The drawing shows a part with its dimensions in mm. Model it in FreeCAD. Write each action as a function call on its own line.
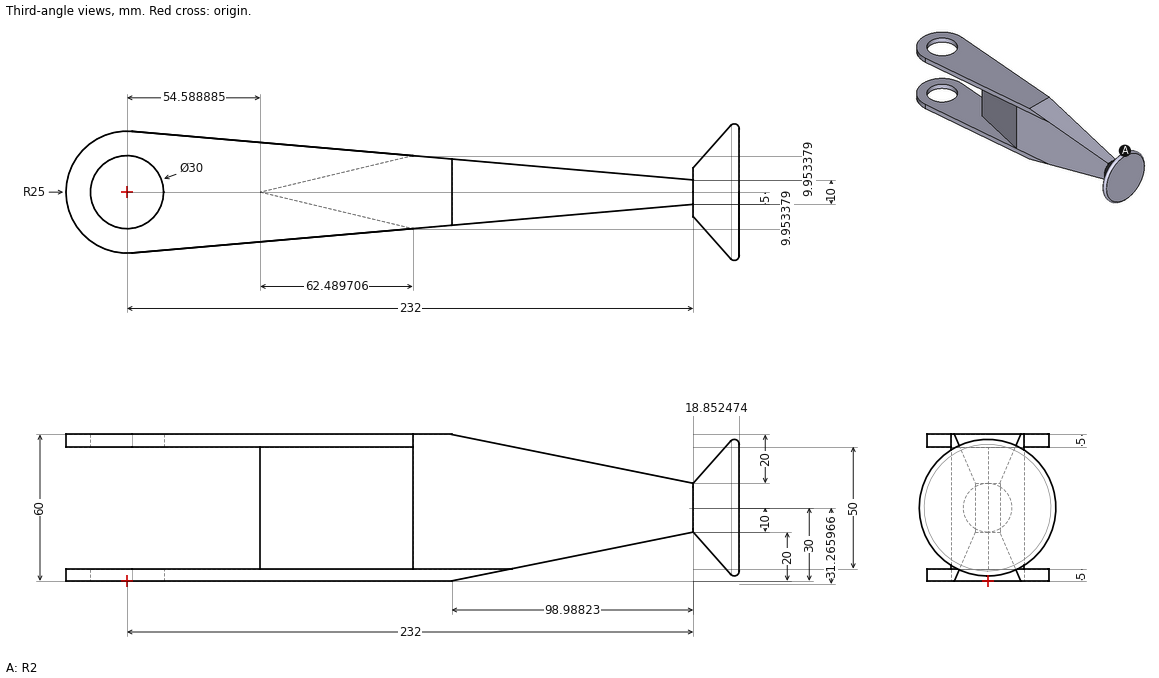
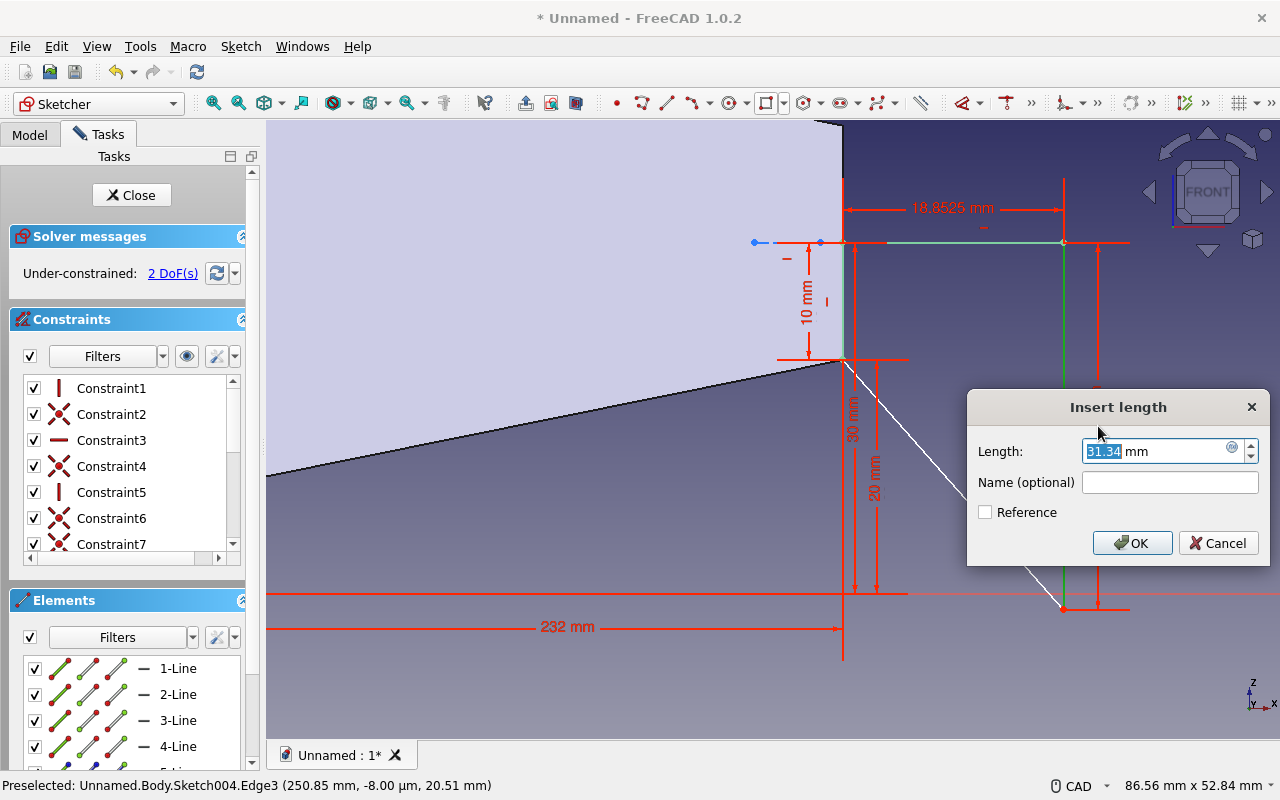
text(31.265966)
key(Return)
key(Escape)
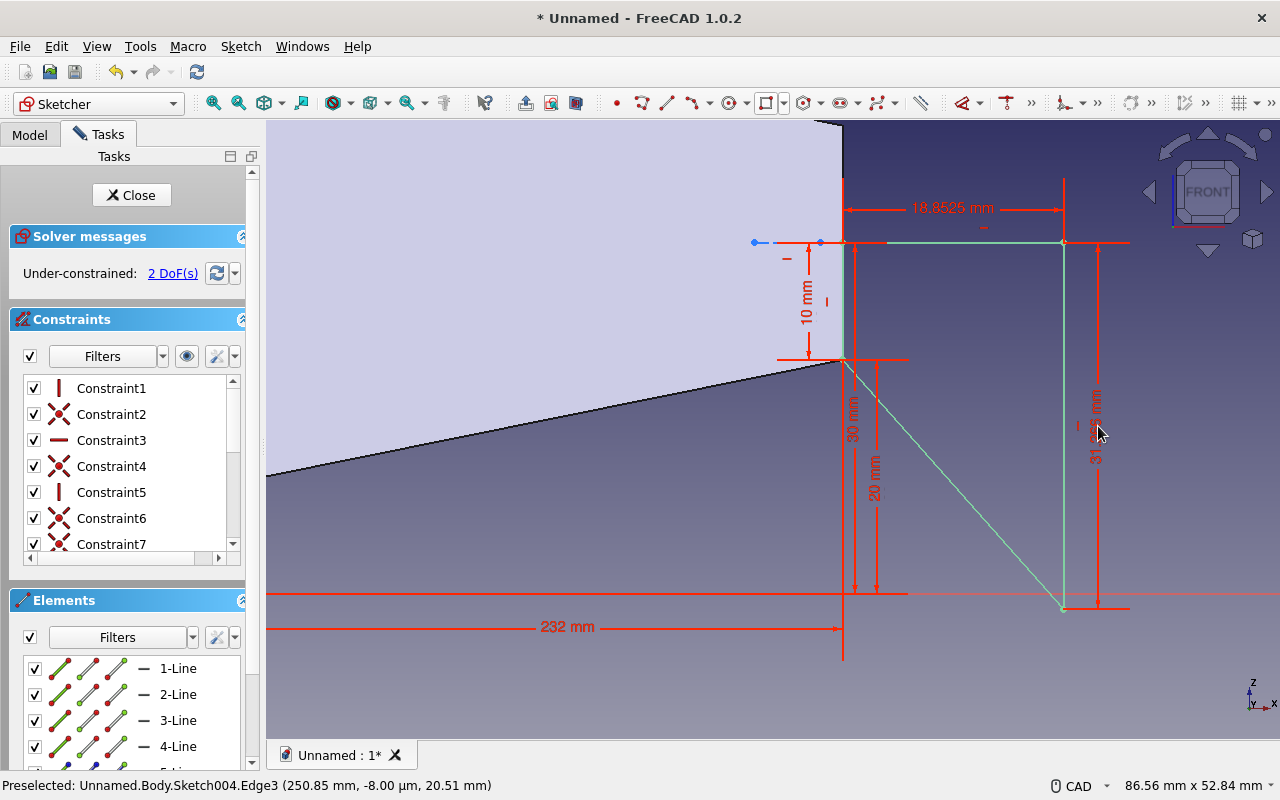
click(132, 195)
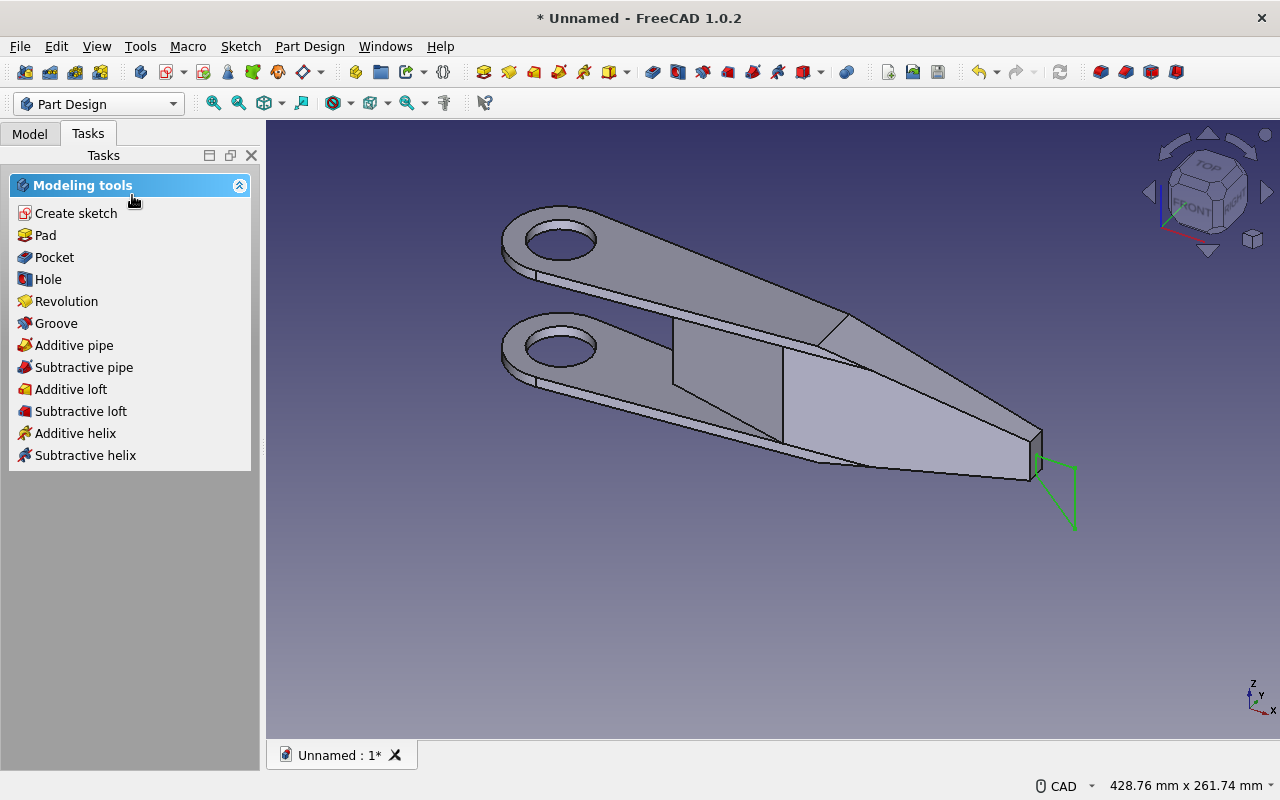
click(509, 72)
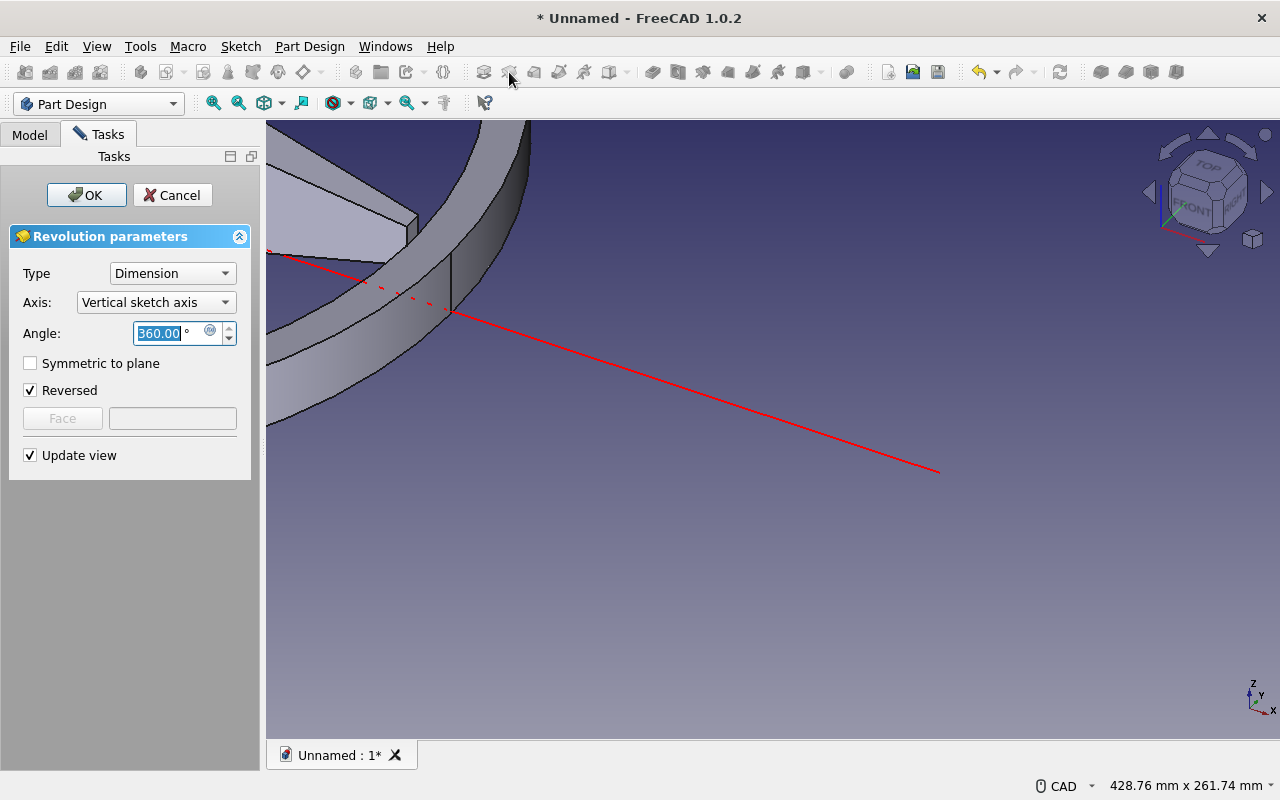
click(157, 302)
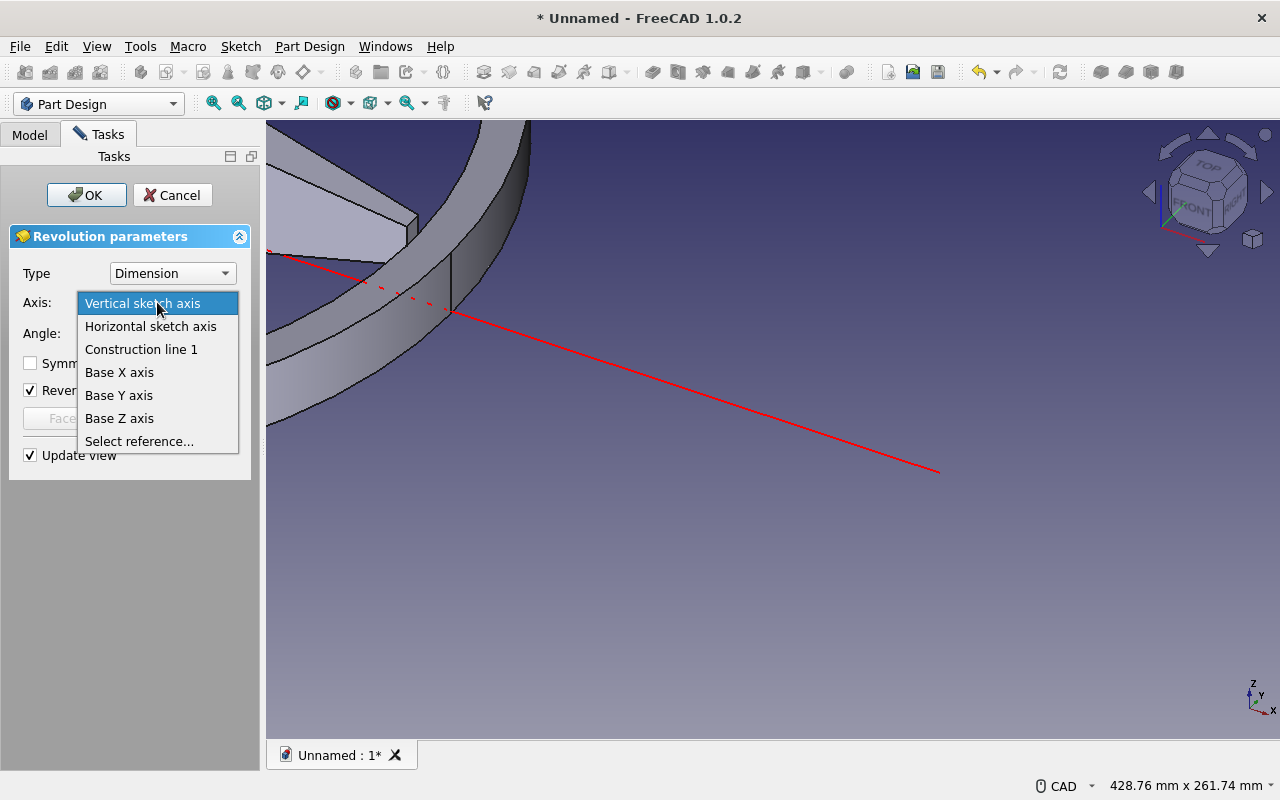
click(156, 350)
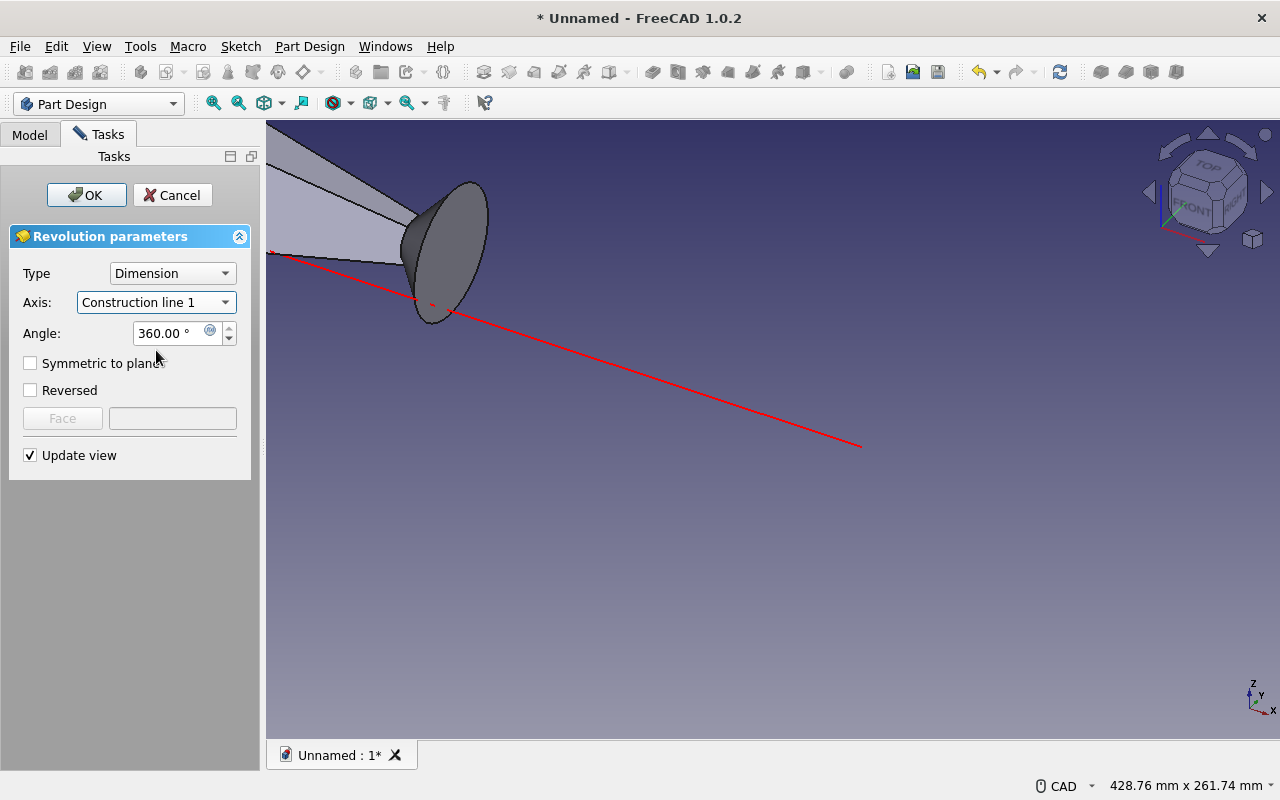
click(87, 195)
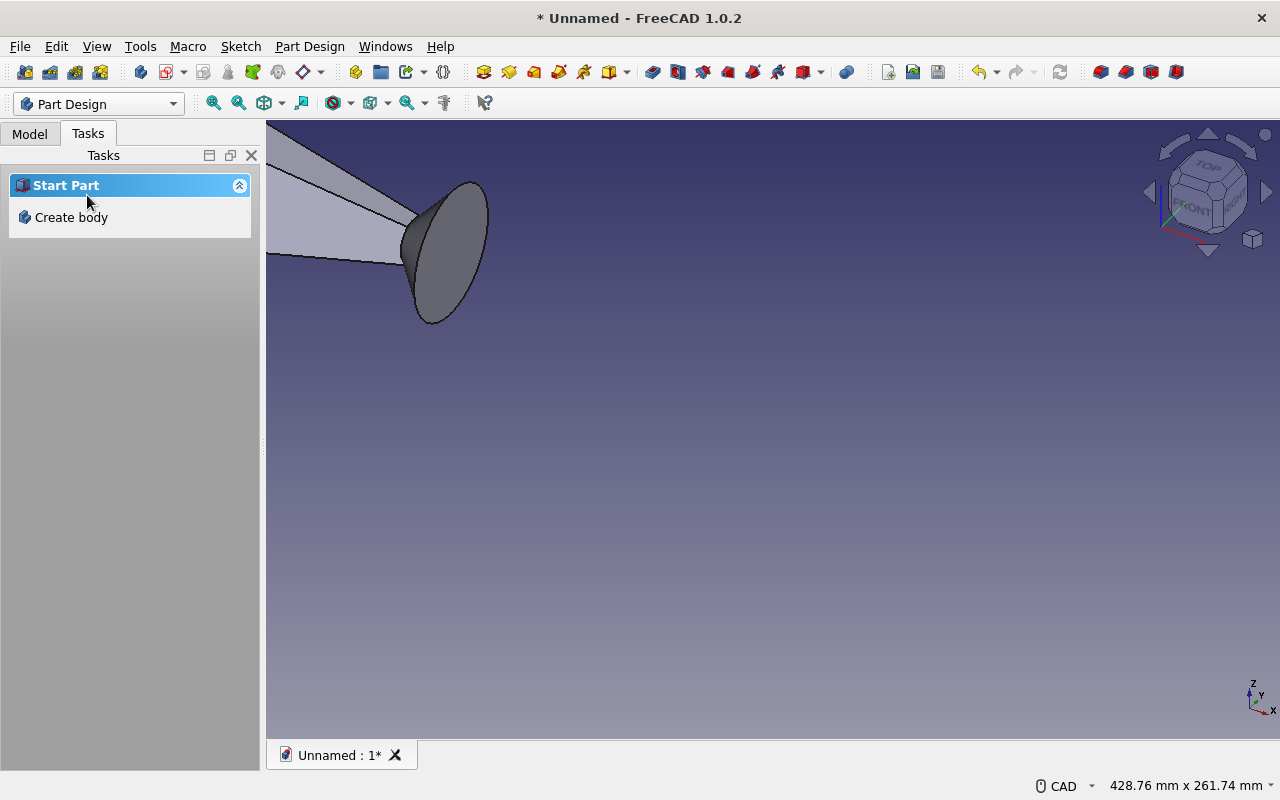
click(214, 104)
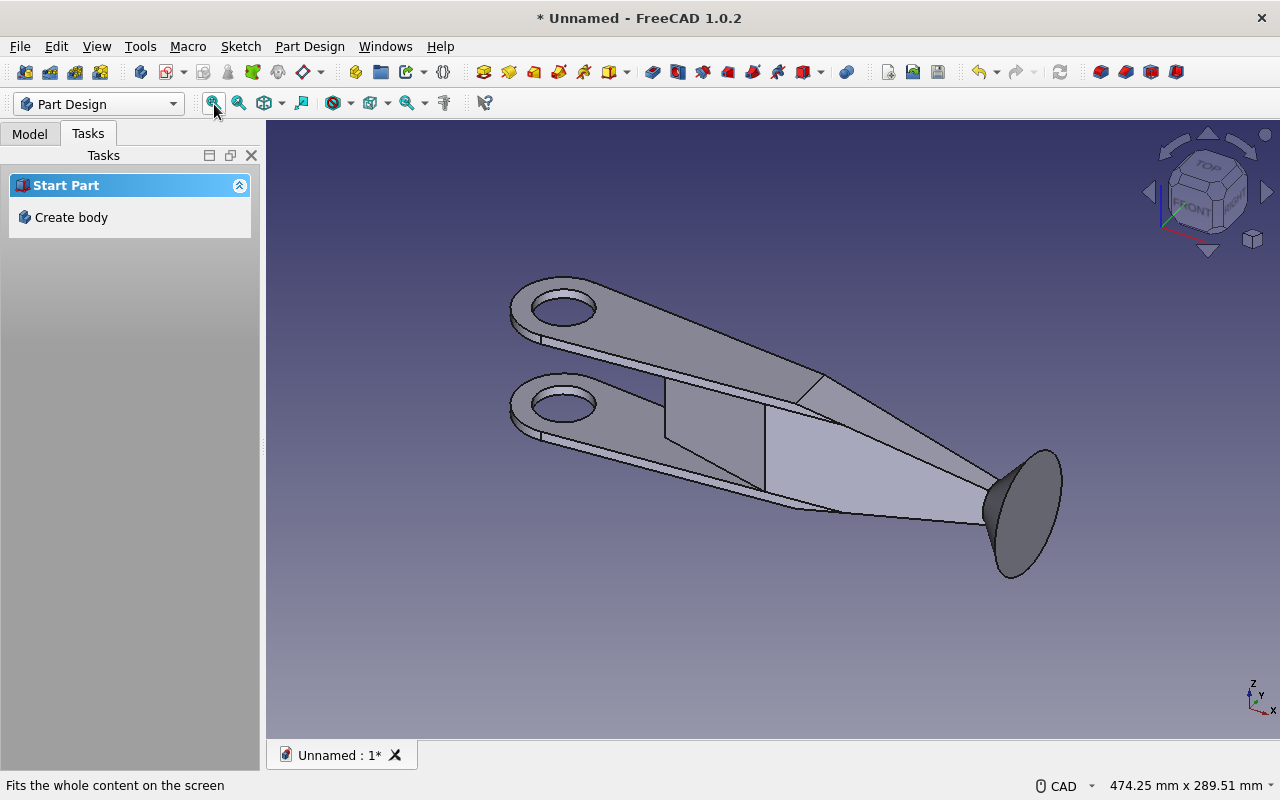
click(1028, 458)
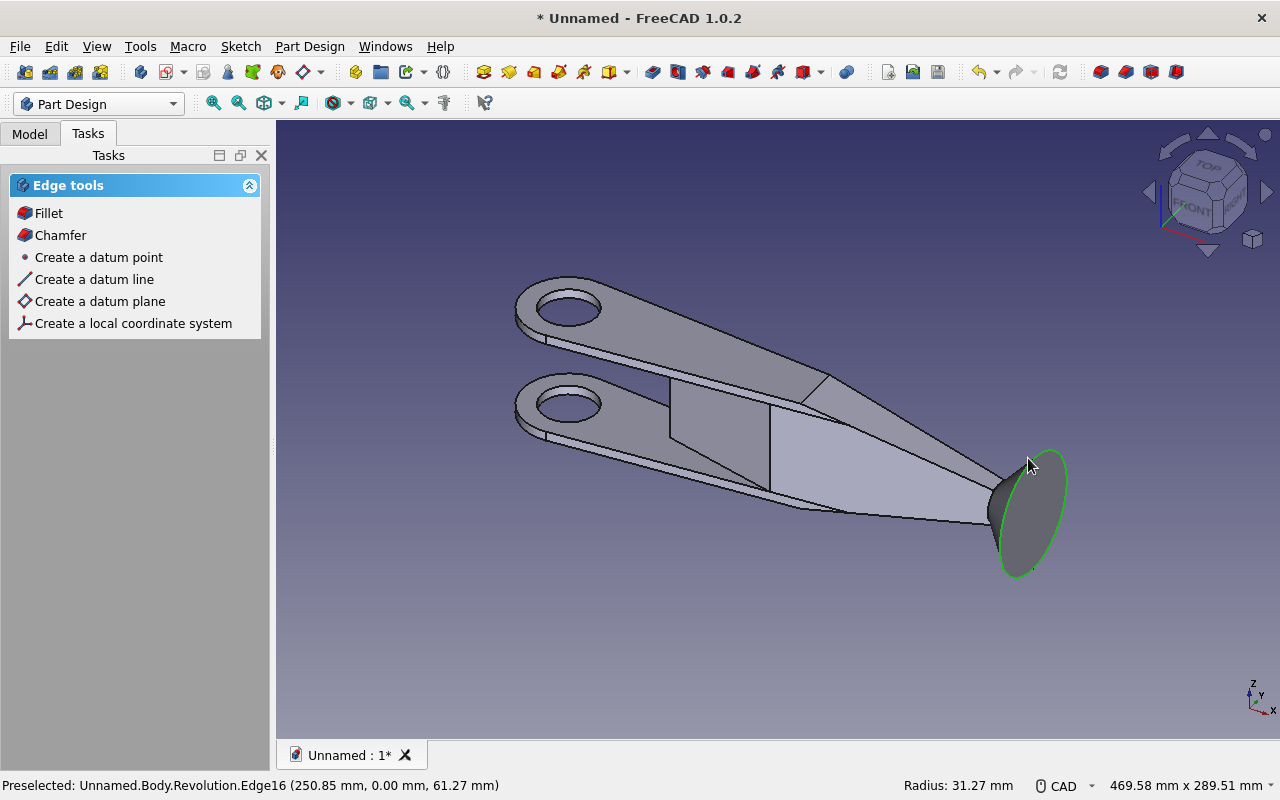
click(1101, 72)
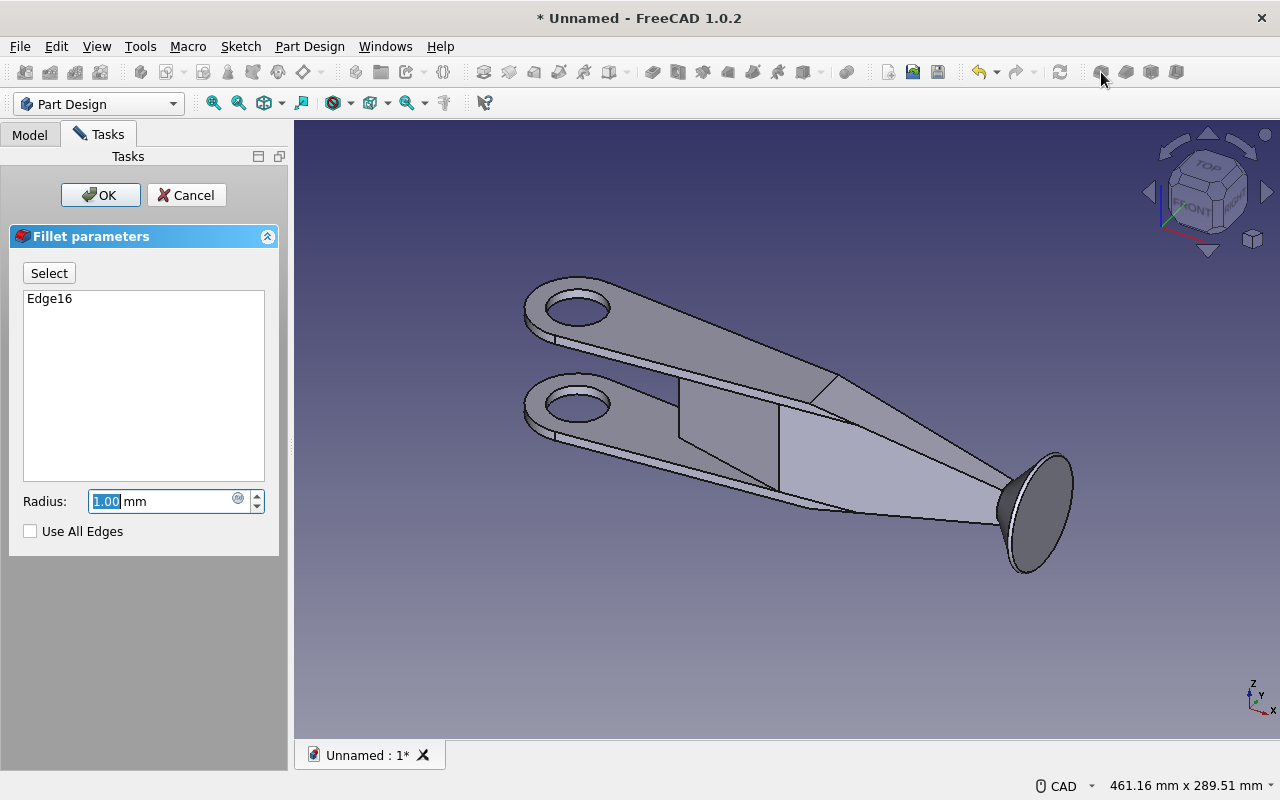
text(2)
key(Tab)